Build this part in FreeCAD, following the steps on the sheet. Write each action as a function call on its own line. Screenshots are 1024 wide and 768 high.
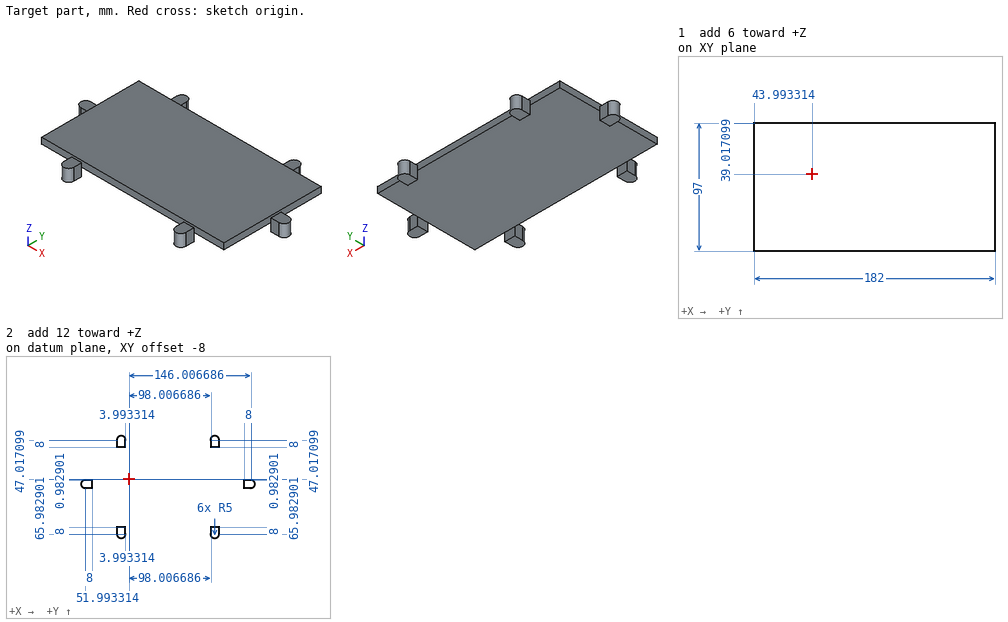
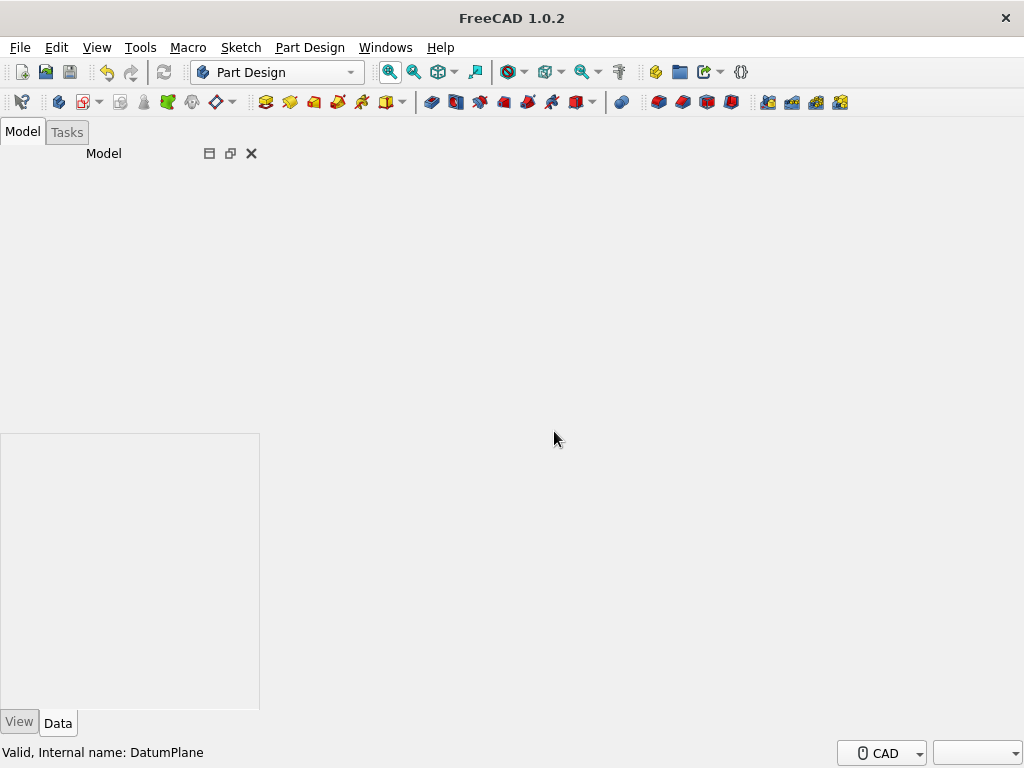
click(22, 72)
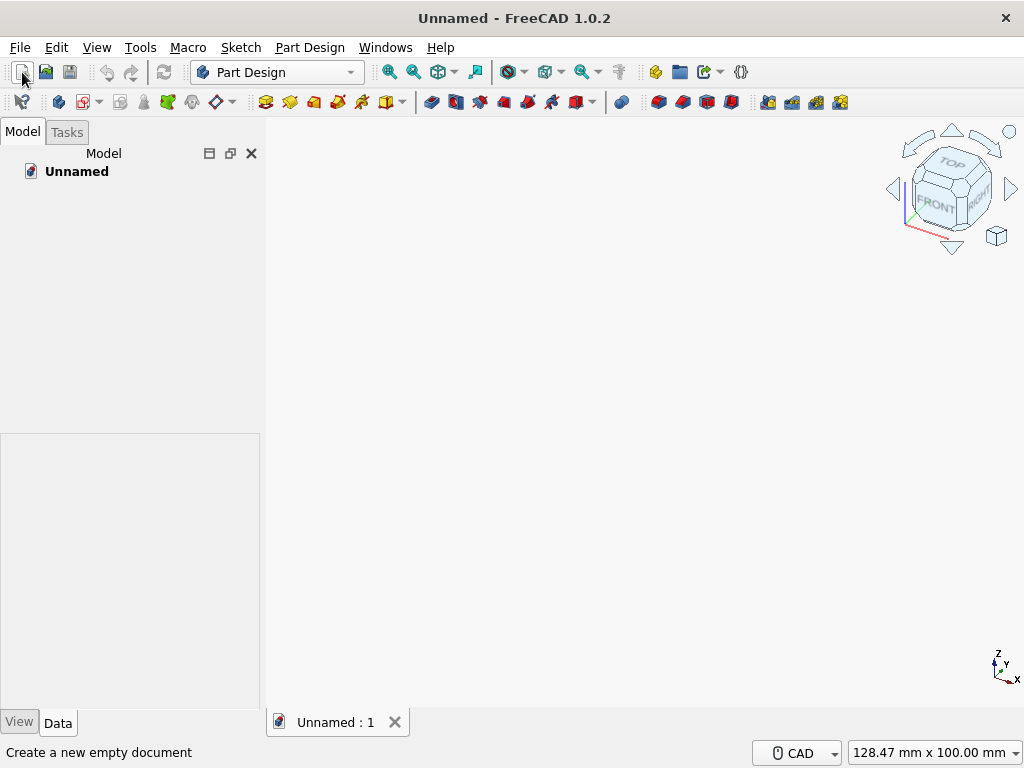
click(84, 102)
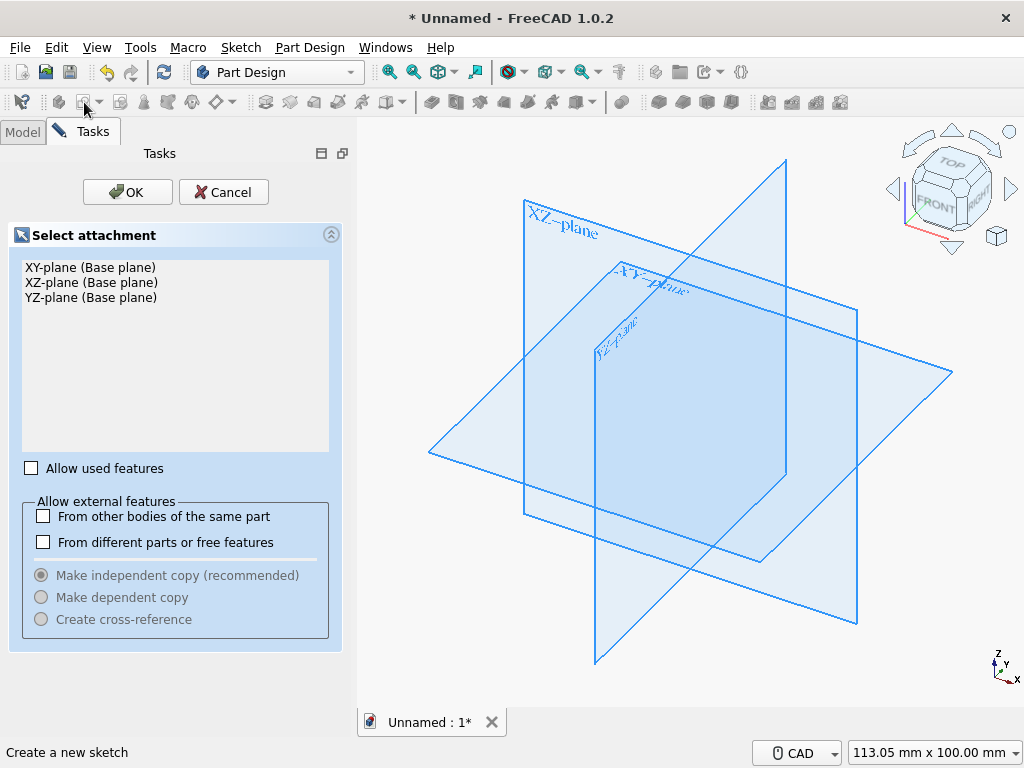
click(82, 268)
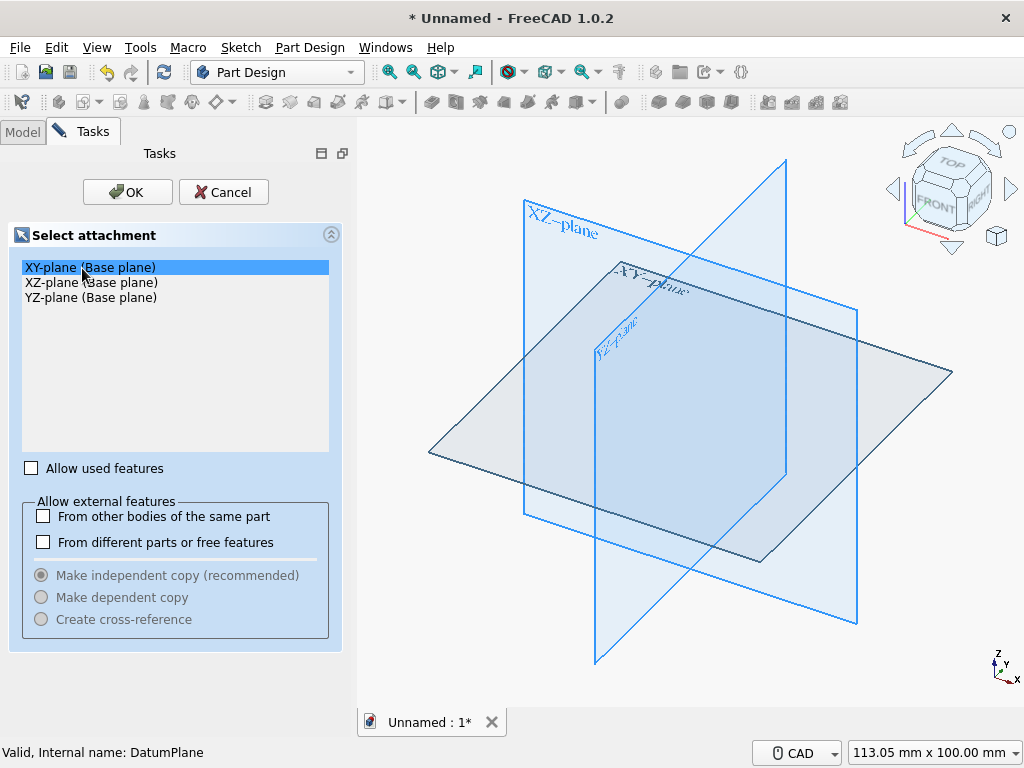
click(128, 192)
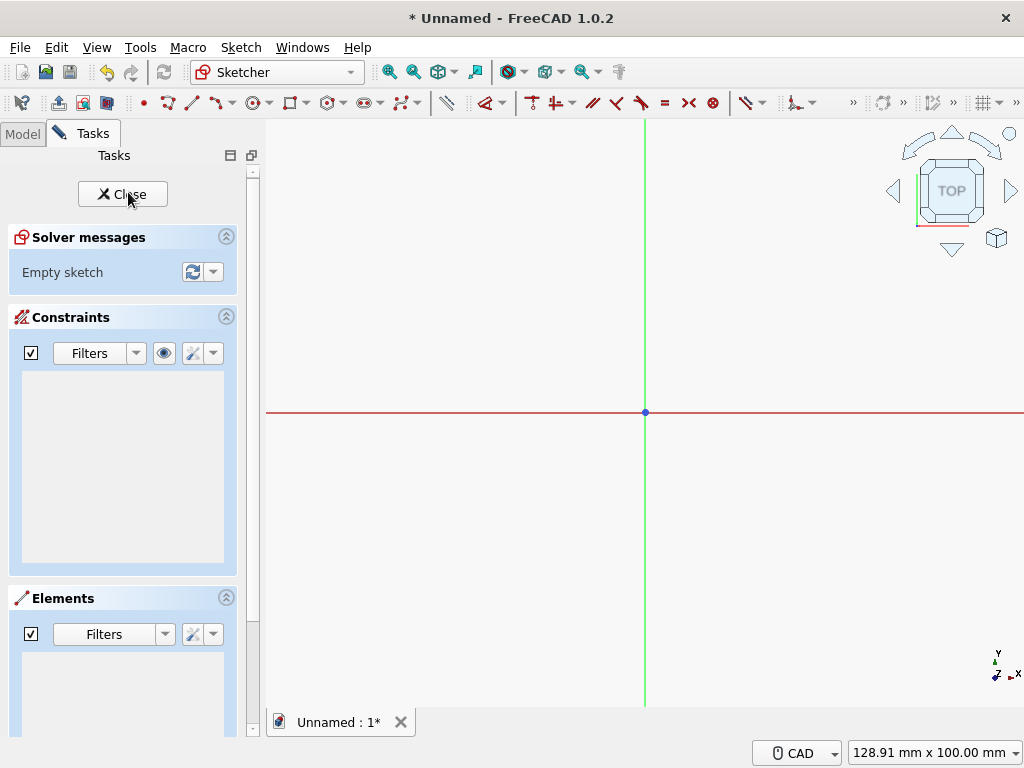
scroll(376, 381, down, 5)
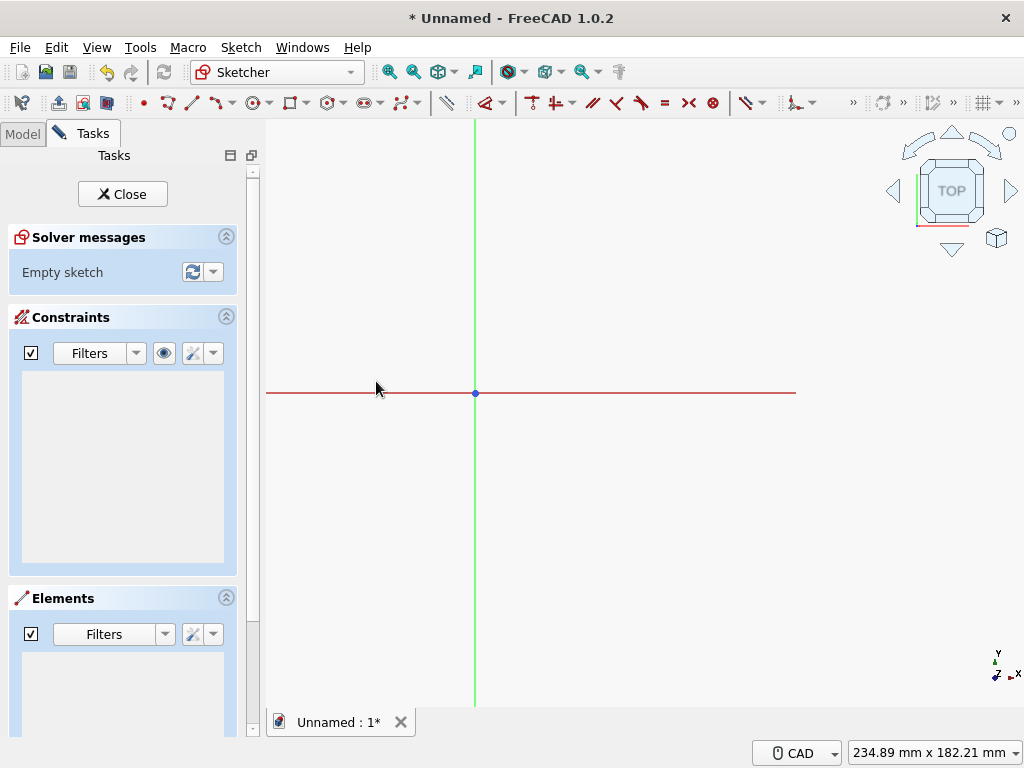
click(290, 104)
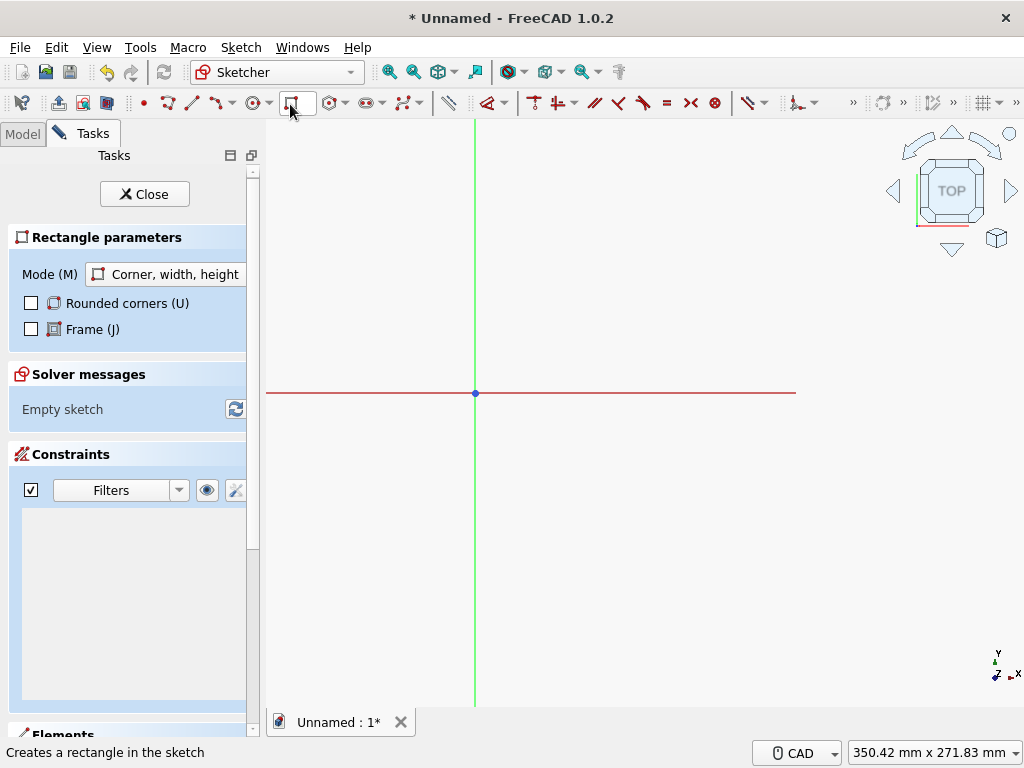
click(380, 309)
click(774, 518)
key(Escape)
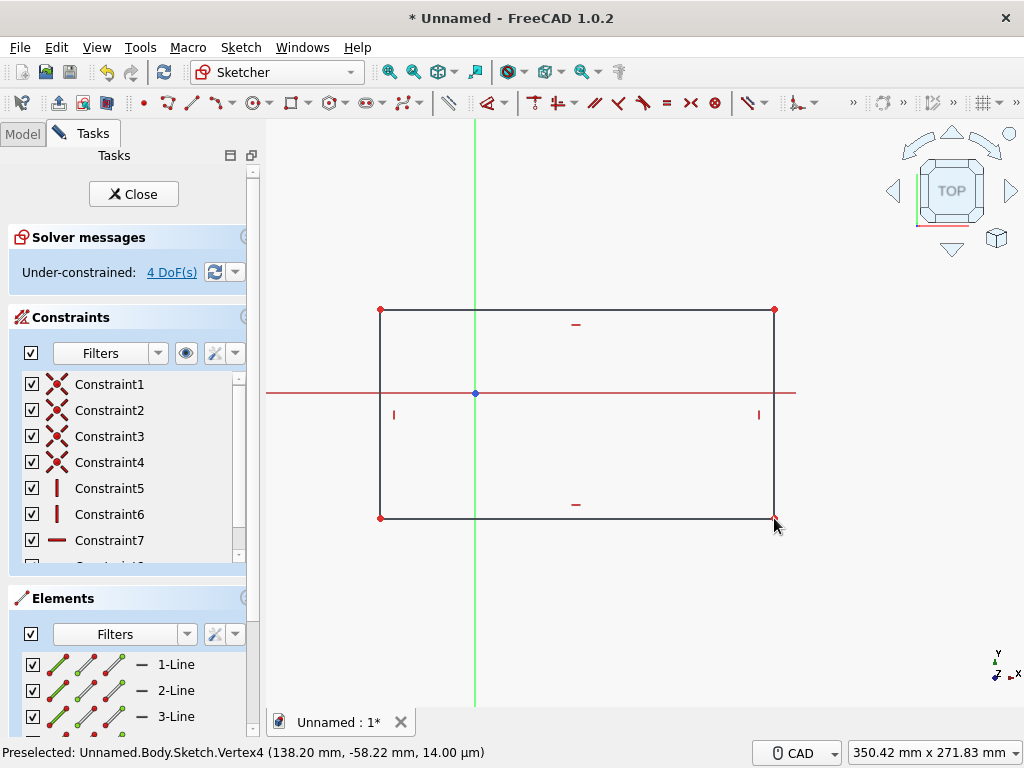
click(488, 104)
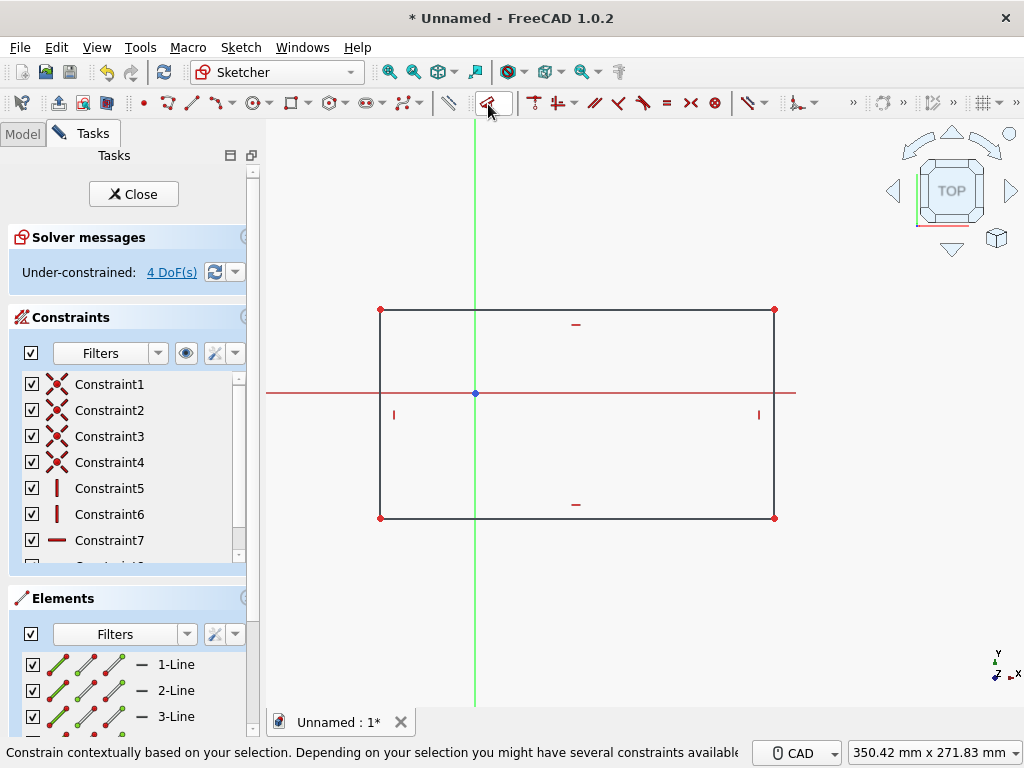
click(380, 373)
click(346, 415)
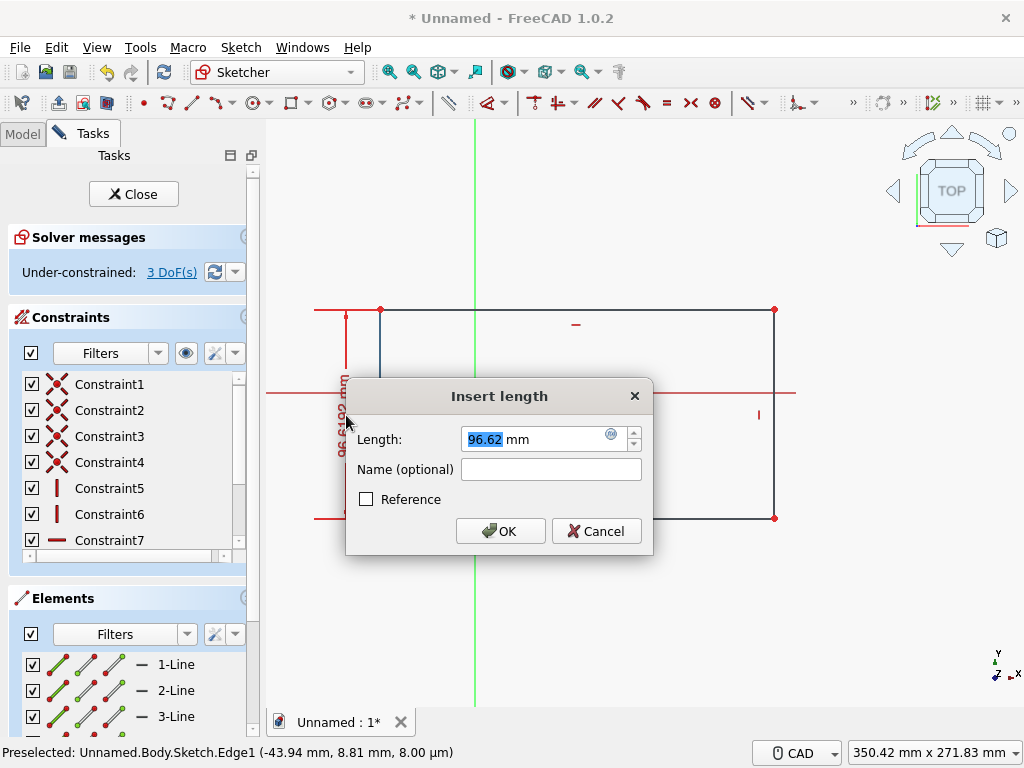
text(97)
key(Return)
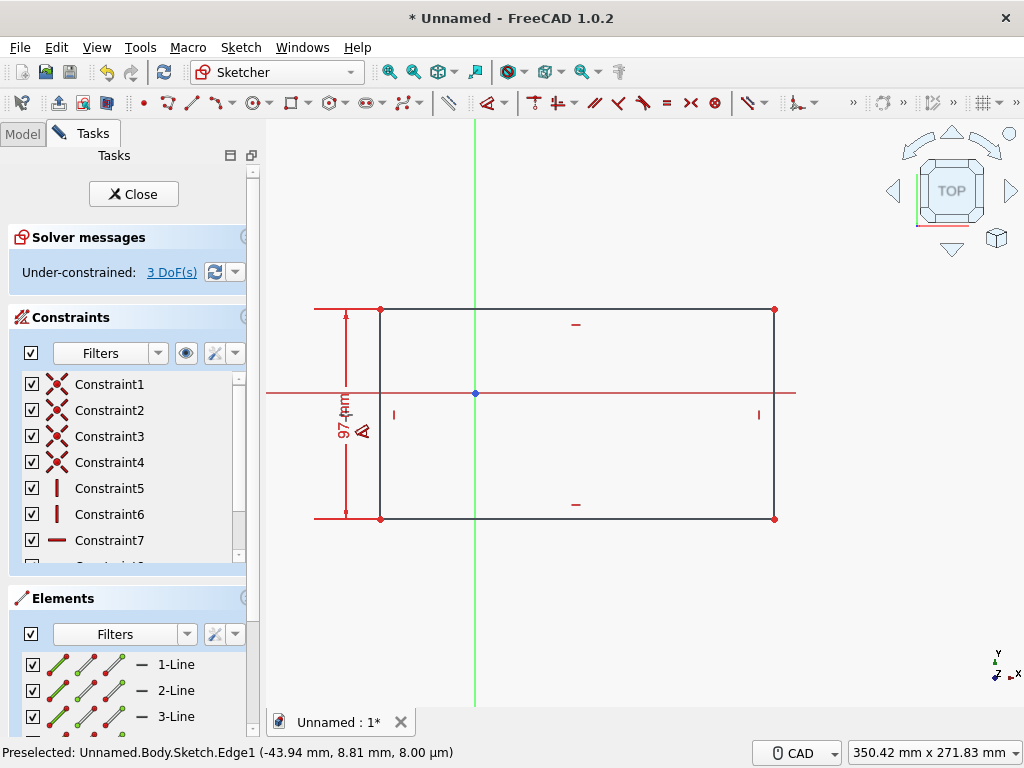
click(498, 519)
click(577, 553)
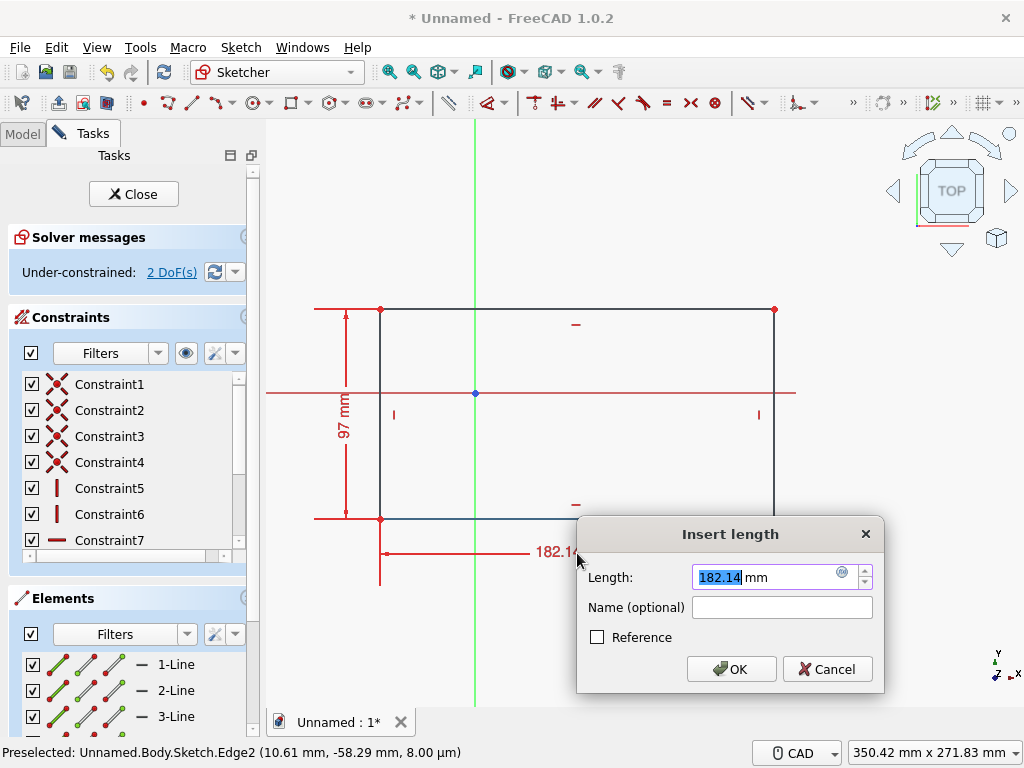
text(182)
key(Return)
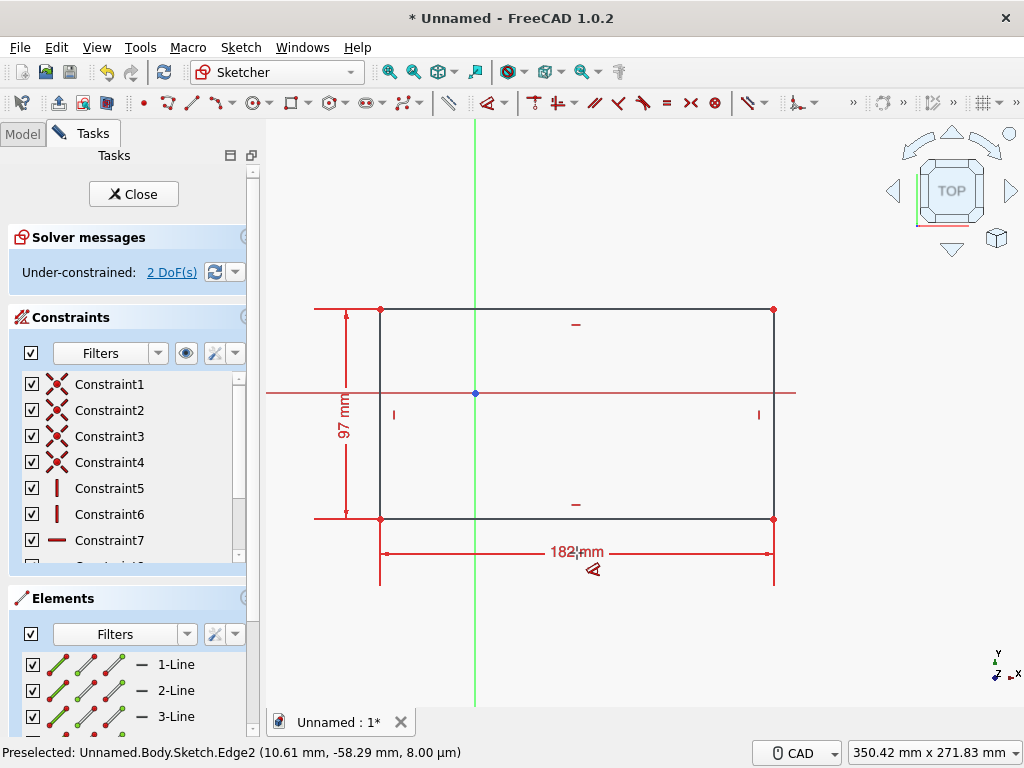
click(380, 309)
click(428, 275)